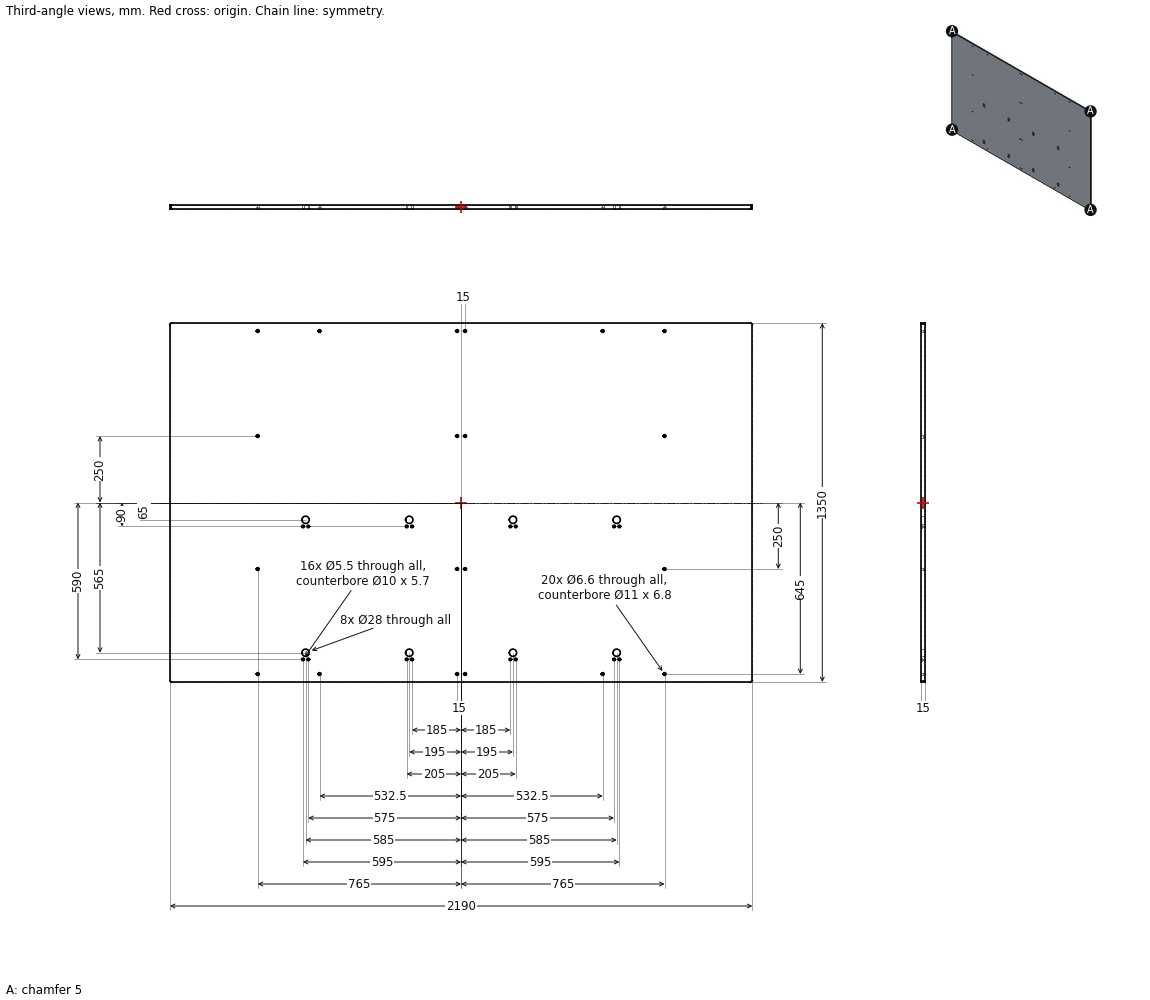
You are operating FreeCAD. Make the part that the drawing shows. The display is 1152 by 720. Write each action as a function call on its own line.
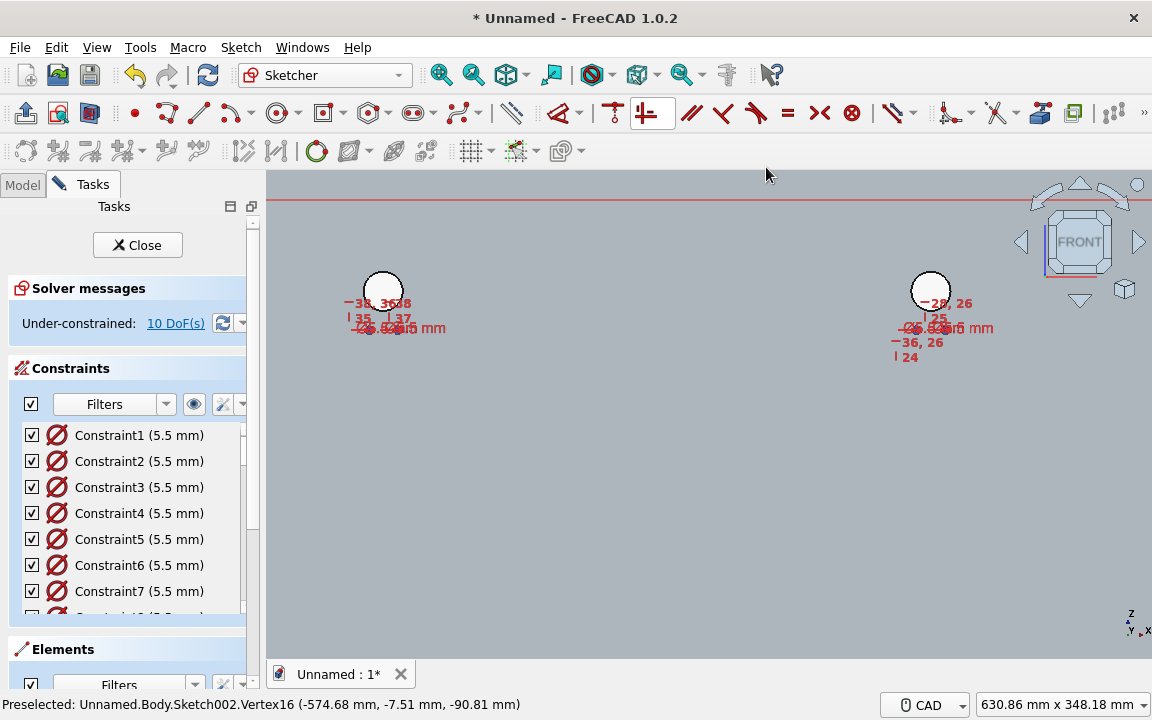
click(916, 330)
click(882, 265)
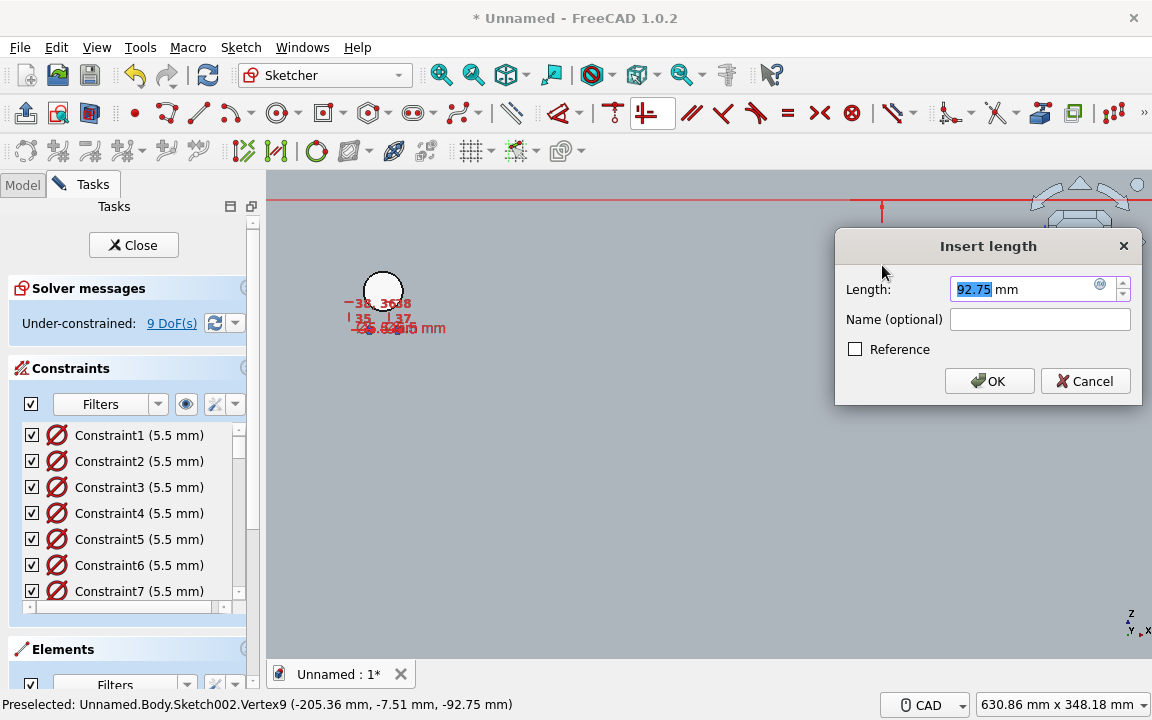
text(90)
key(Return)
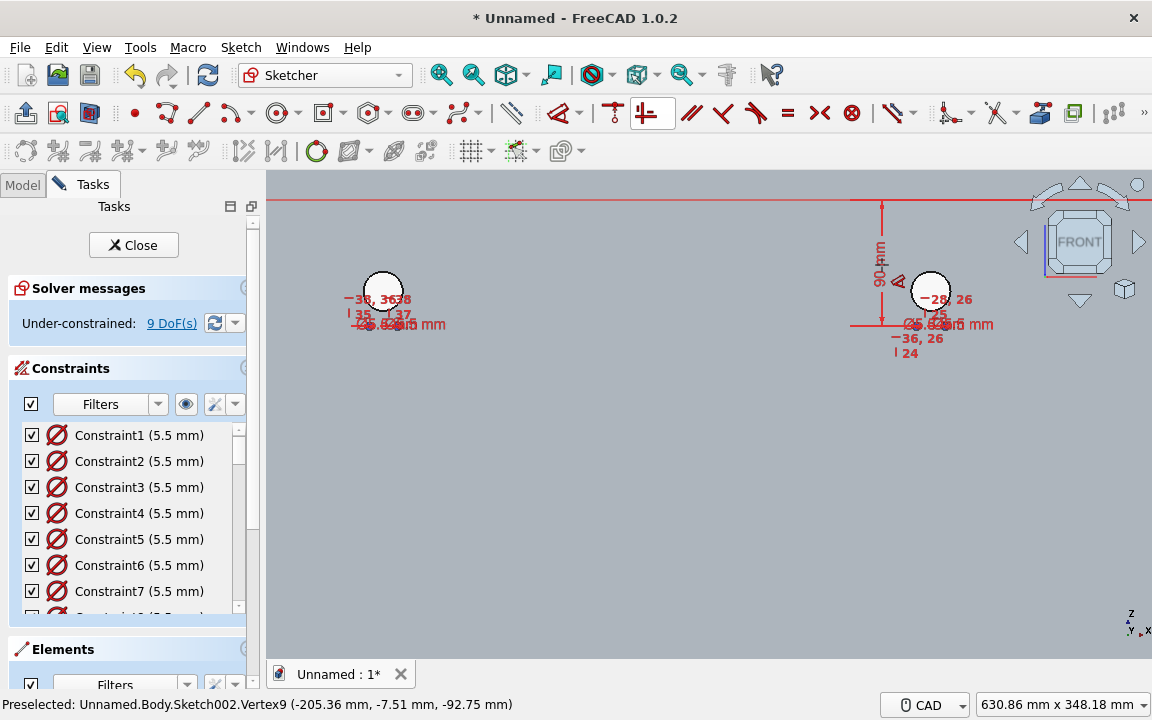
scroll(397, 328, down, 6)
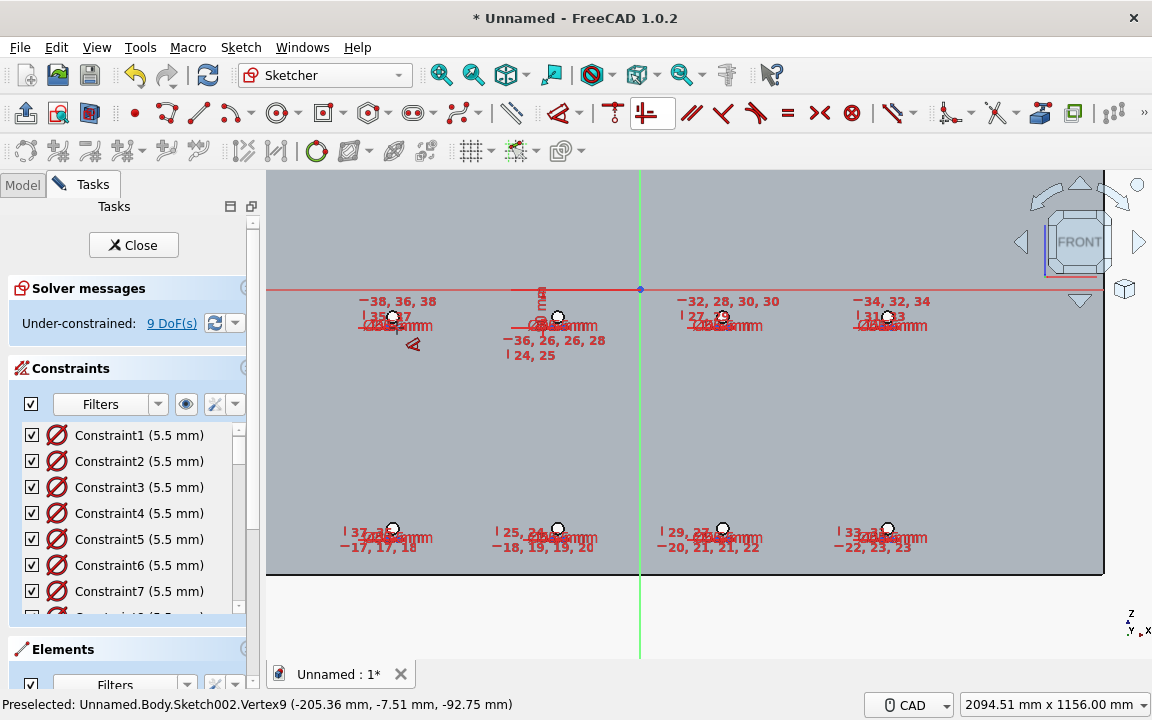
scroll(389, 540, up, 2)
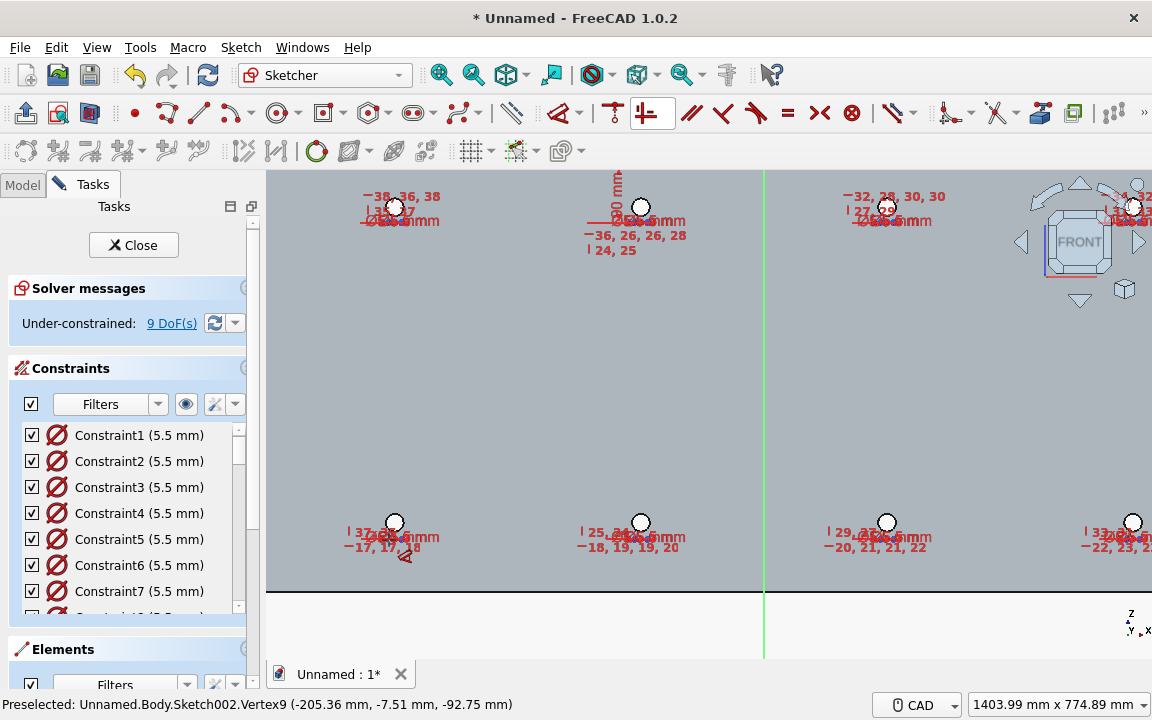
click(389, 539)
click(576, 573)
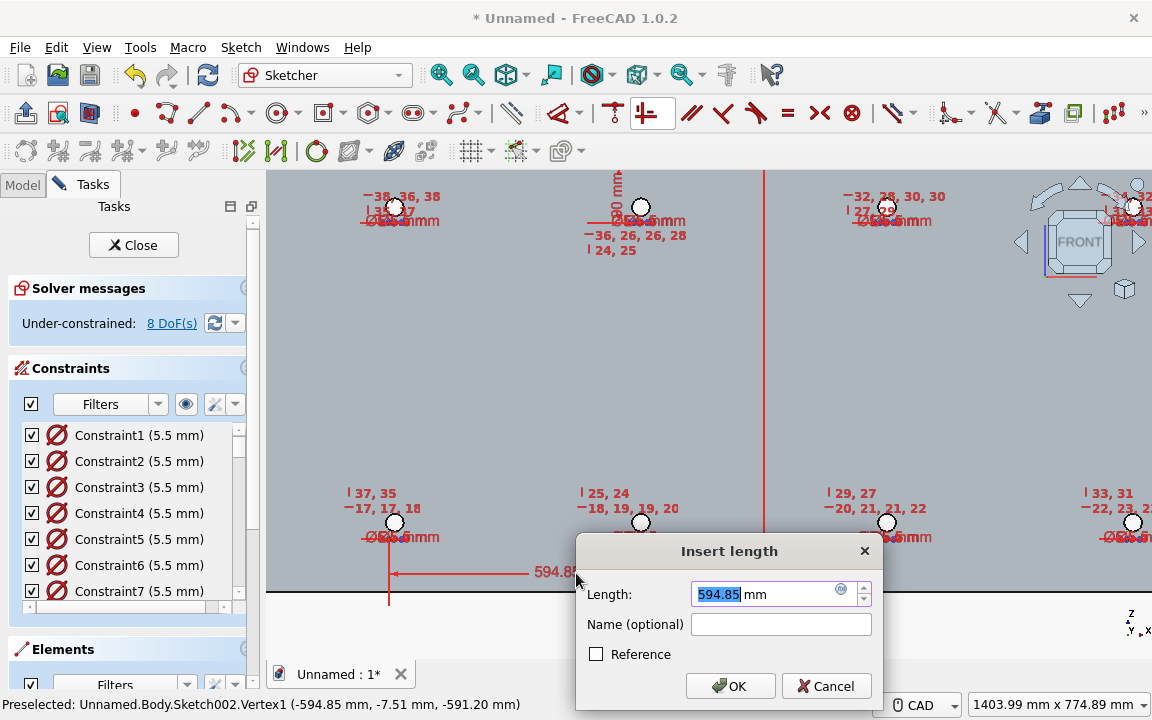
text(595)
key(Return)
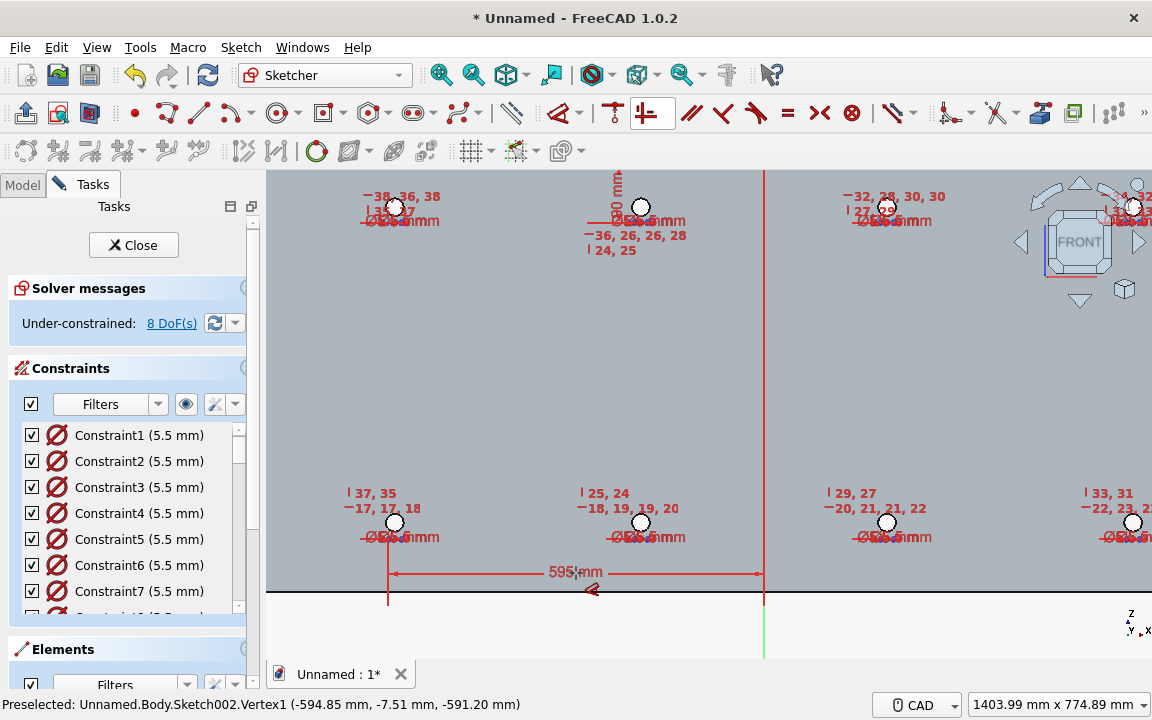
click(389, 539)
click(355, 369)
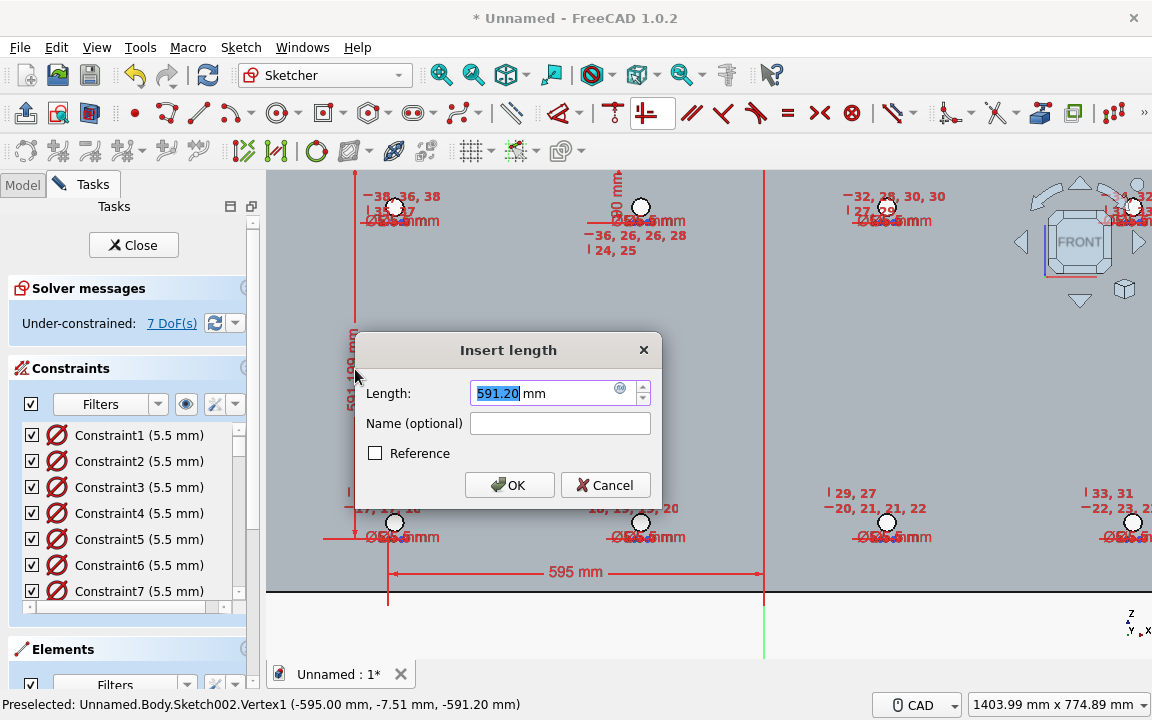
text(590)
key(Return)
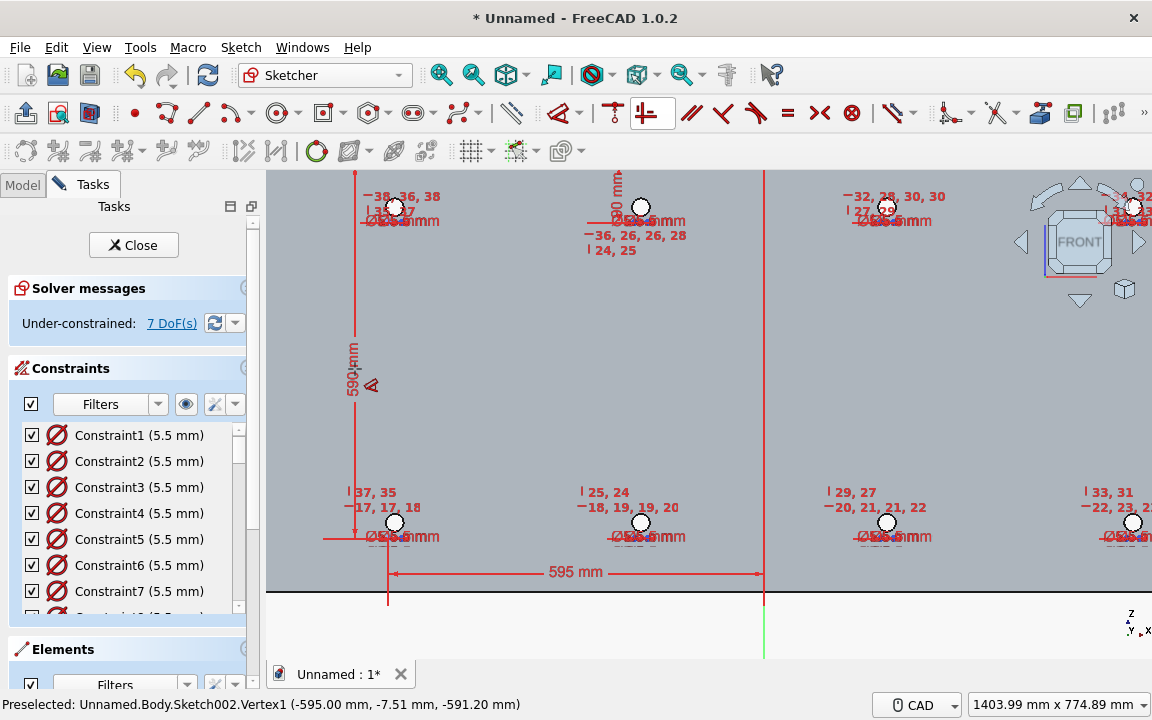
click(401, 539)
click(499, 573)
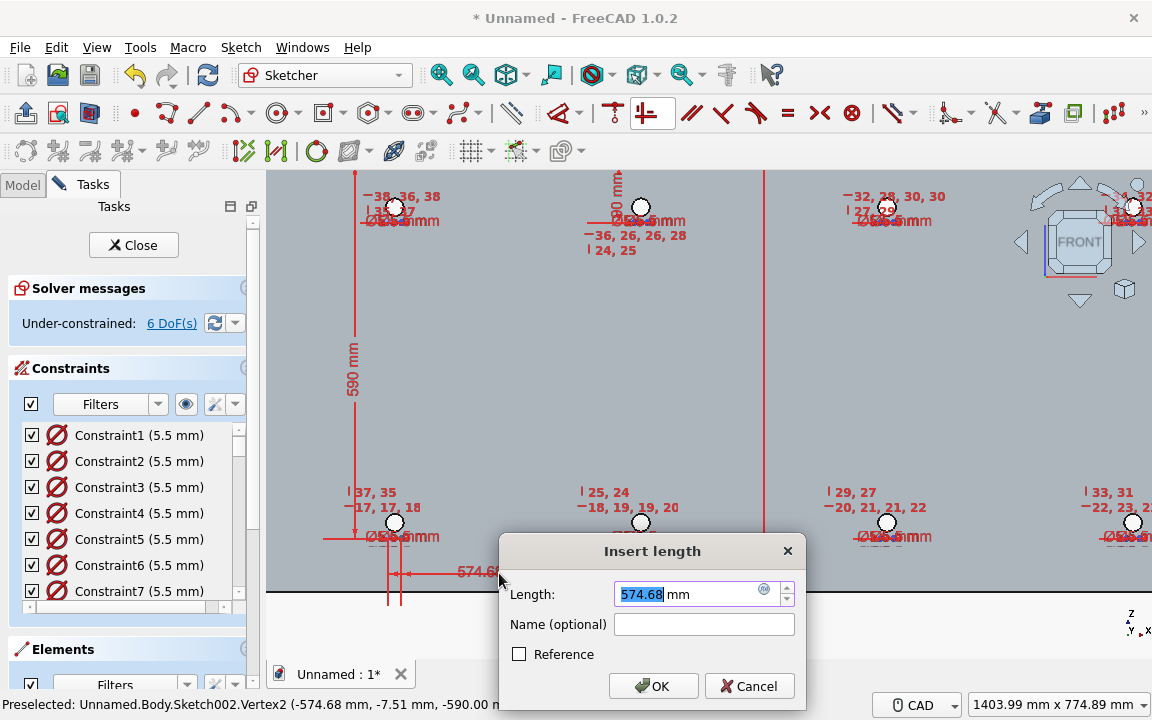
text(575)
key(Return)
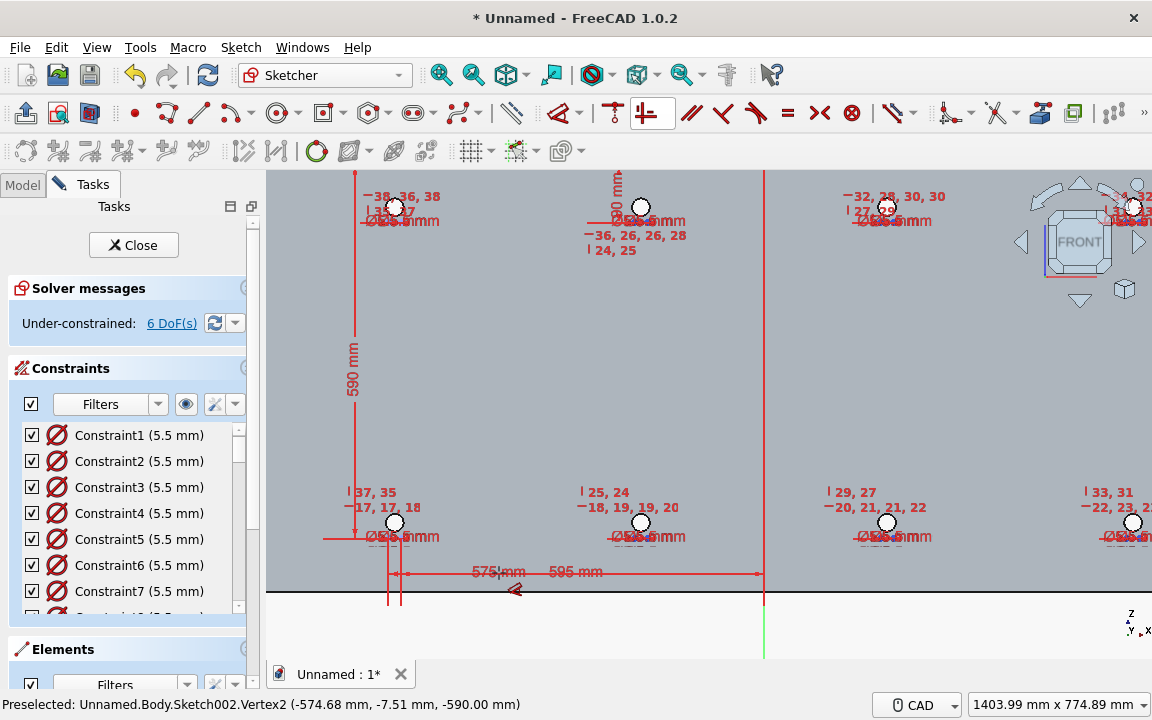
click(634, 539)
click(699, 573)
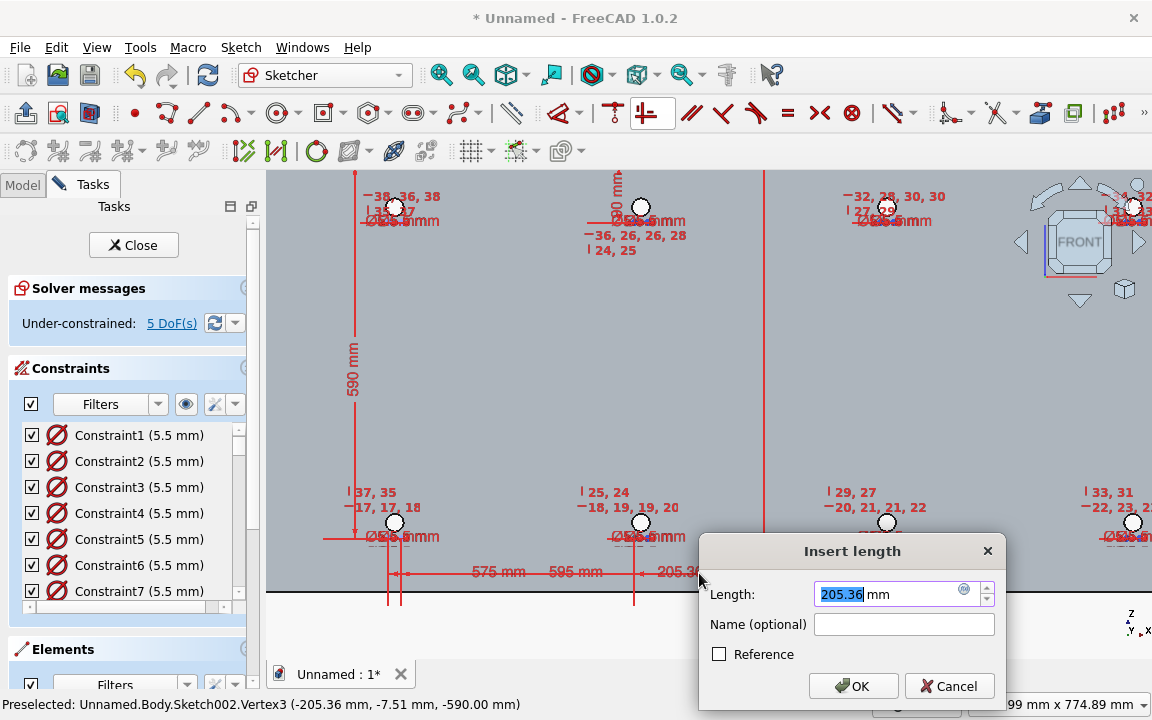
text(205)
key(Return)